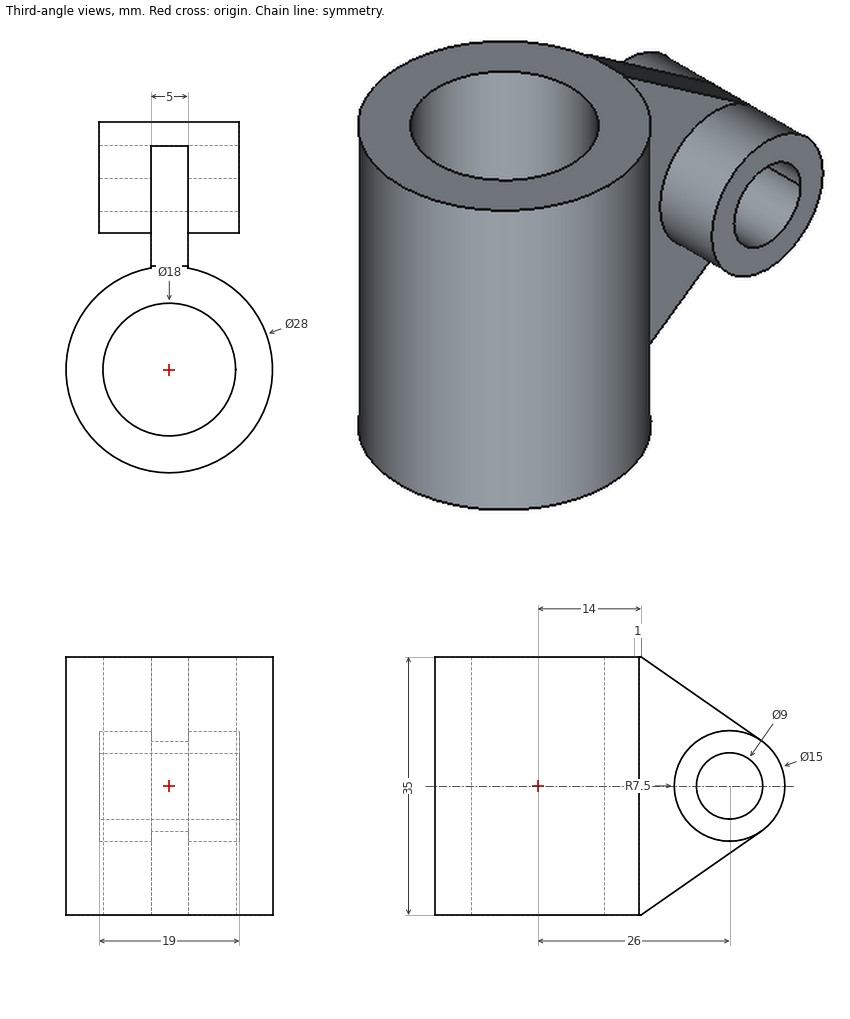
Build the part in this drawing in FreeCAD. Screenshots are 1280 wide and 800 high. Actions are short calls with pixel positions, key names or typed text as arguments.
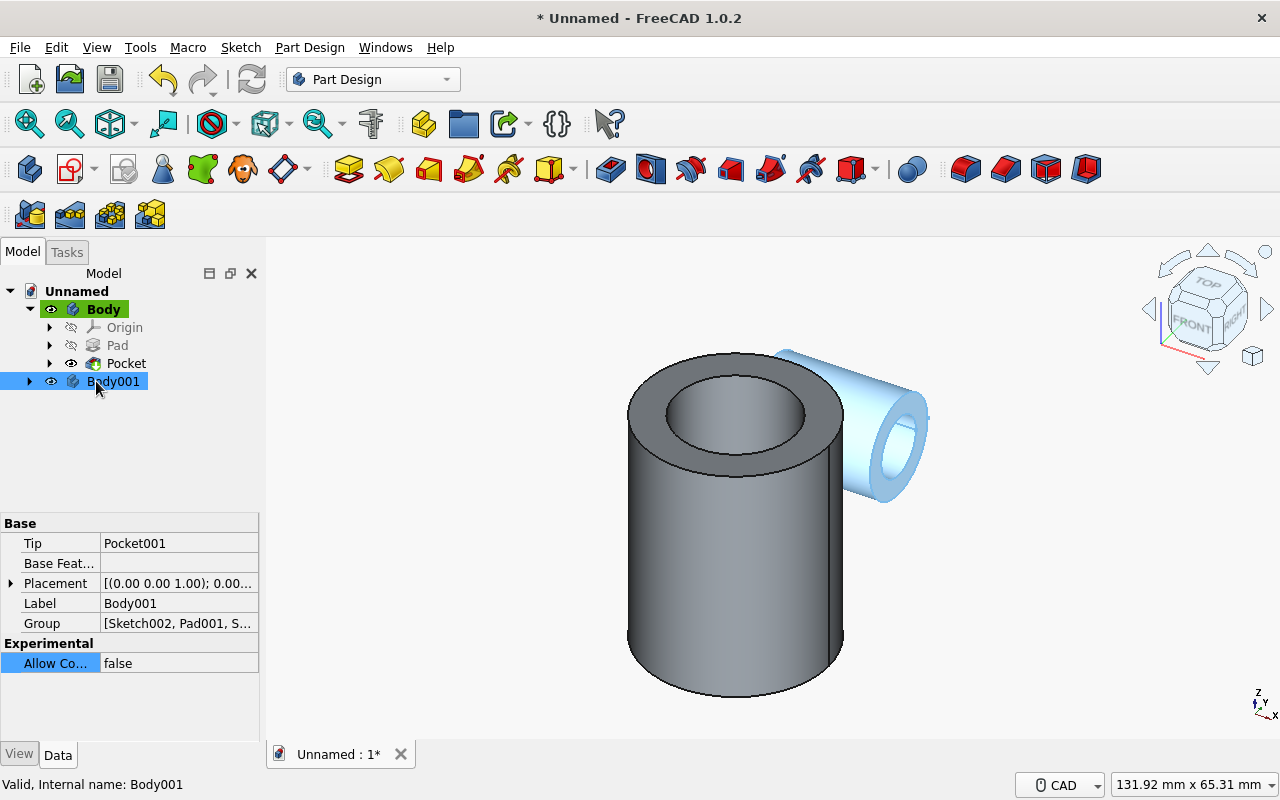
click(914, 170)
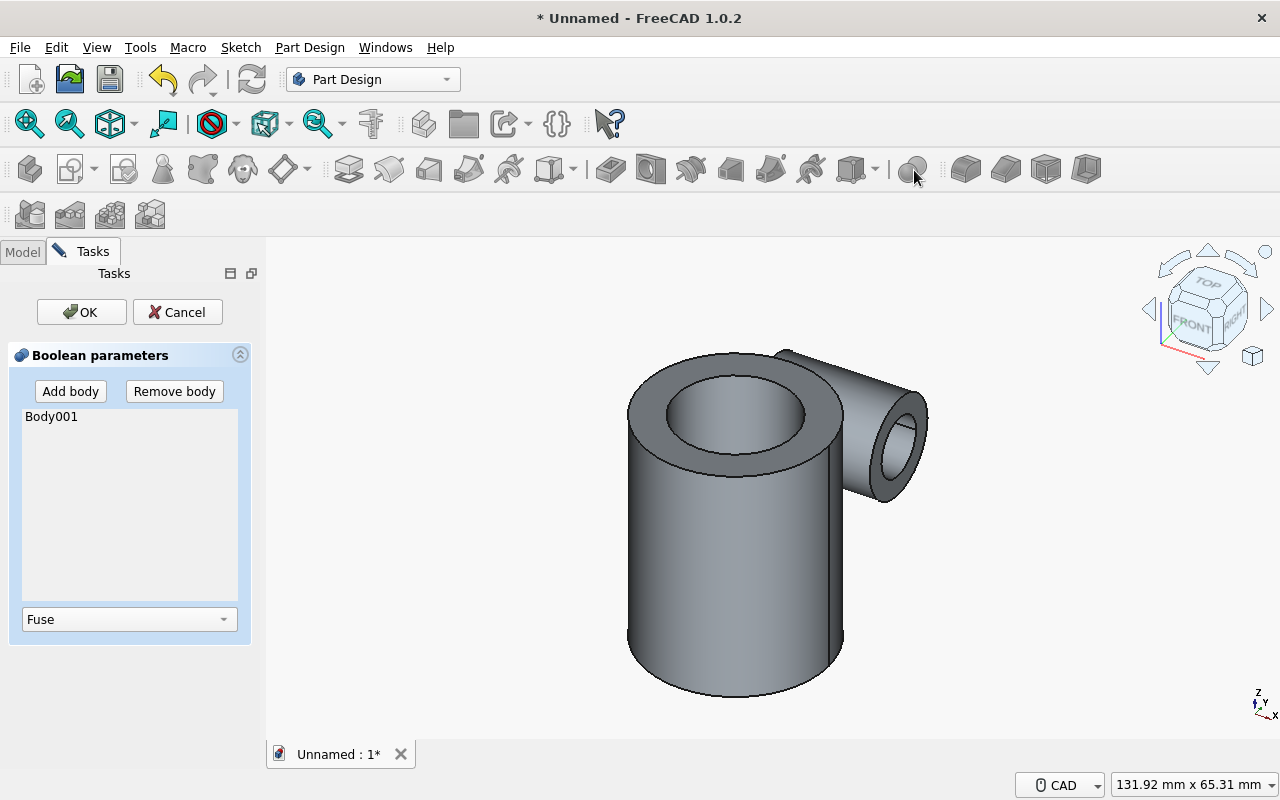
click(82, 312)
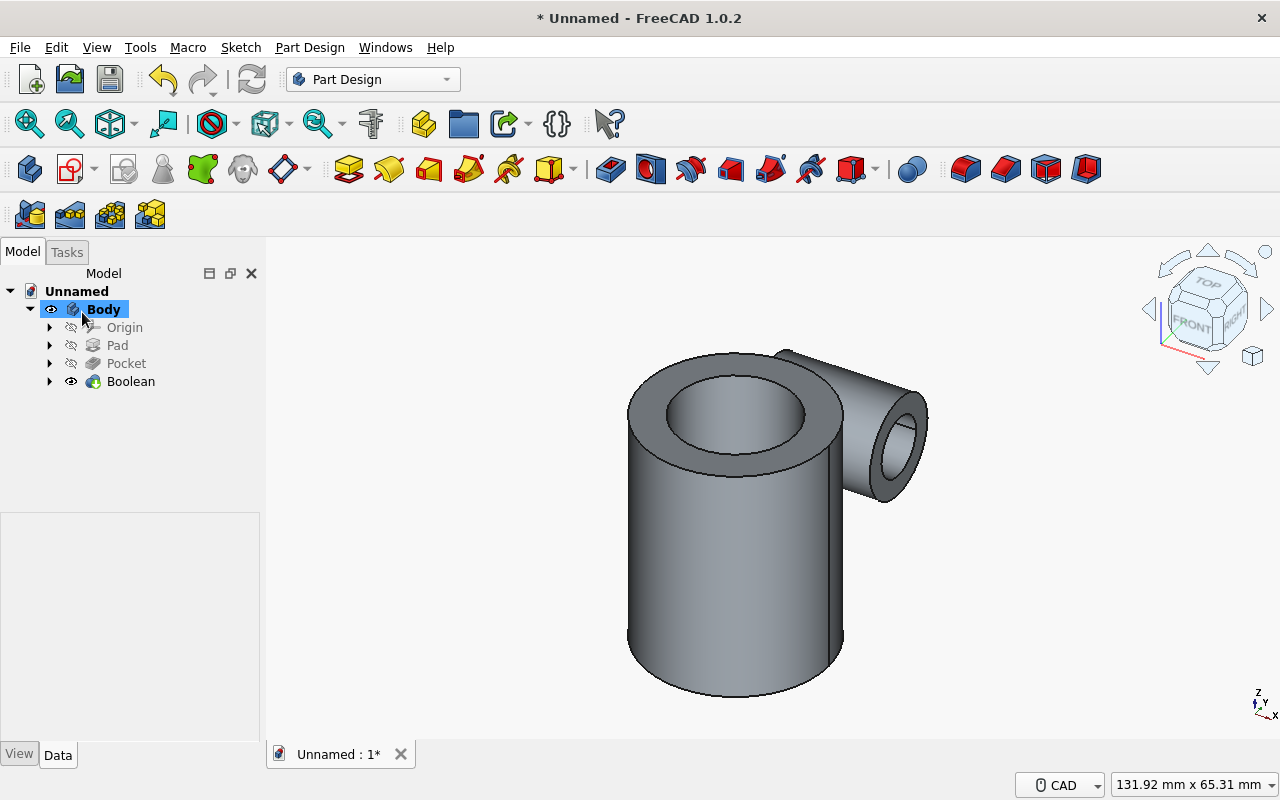
click(70, 170)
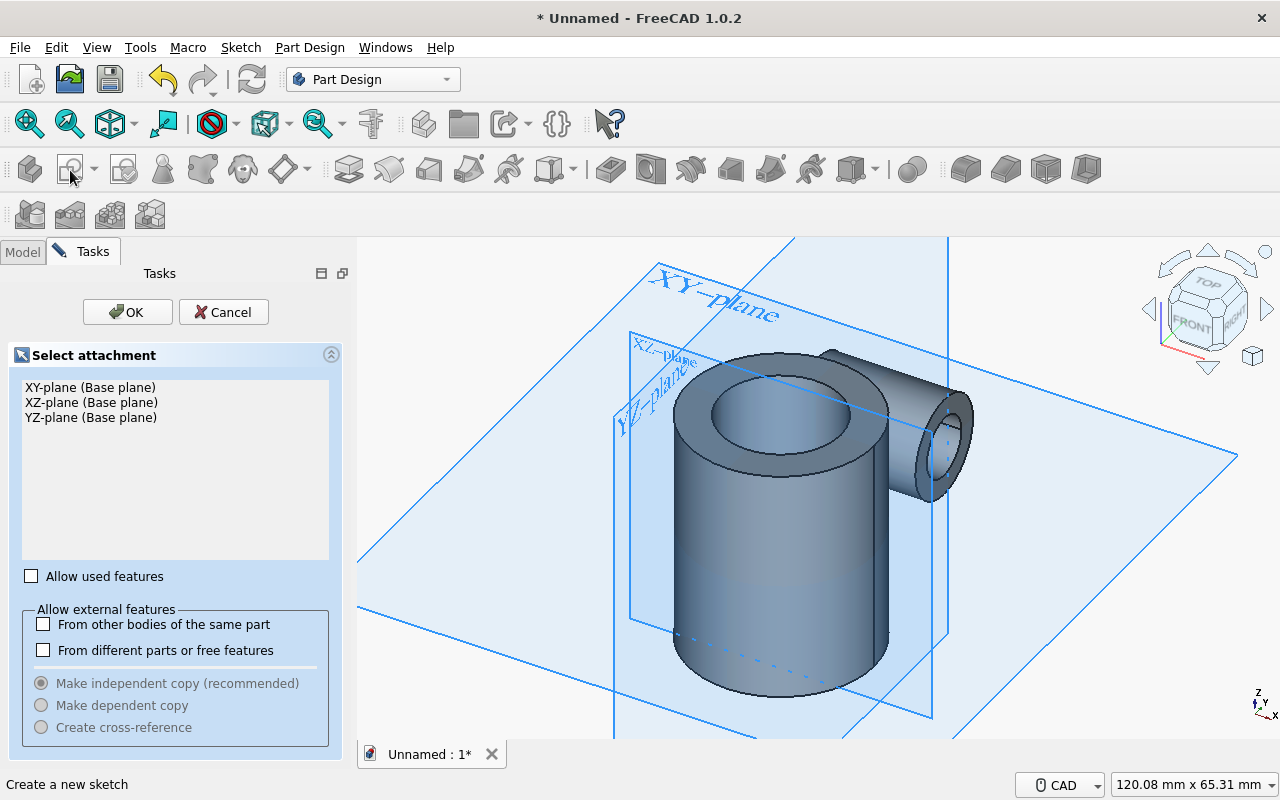
click(82, 418)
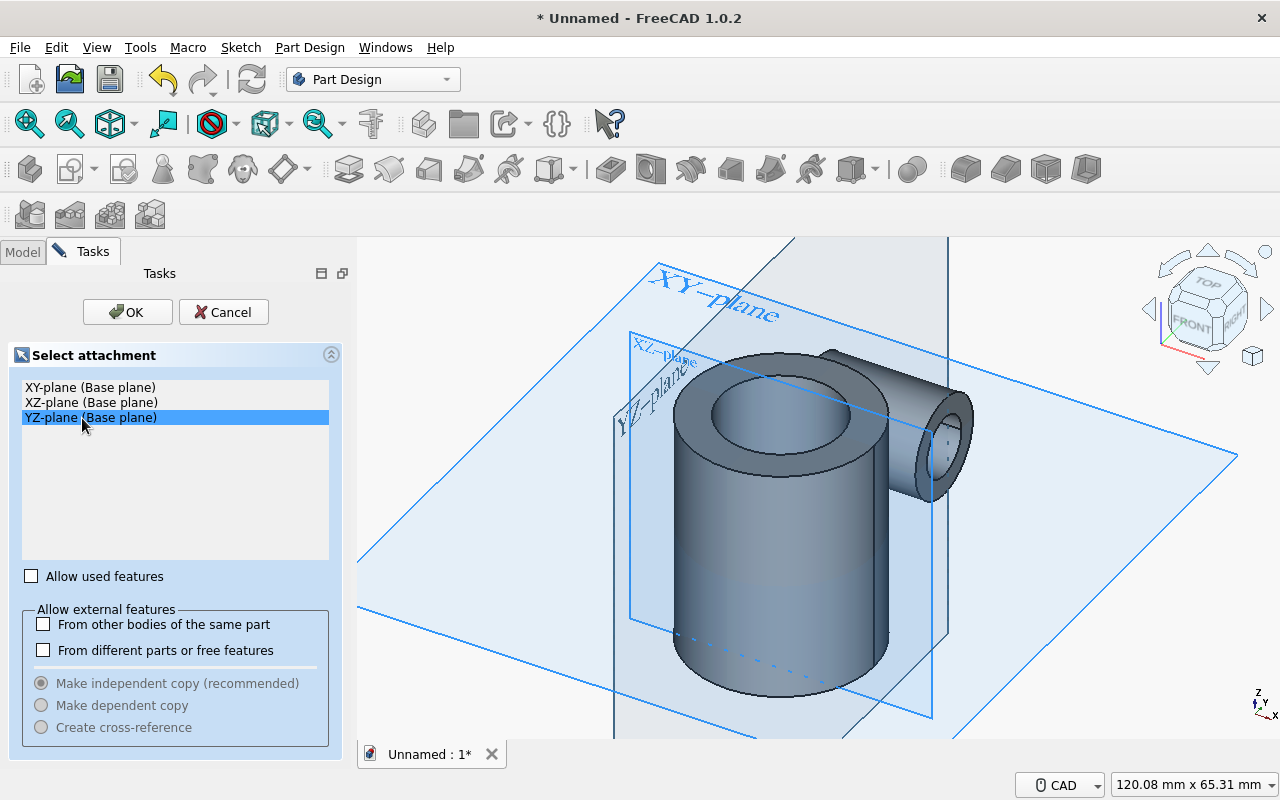
click(128, 312)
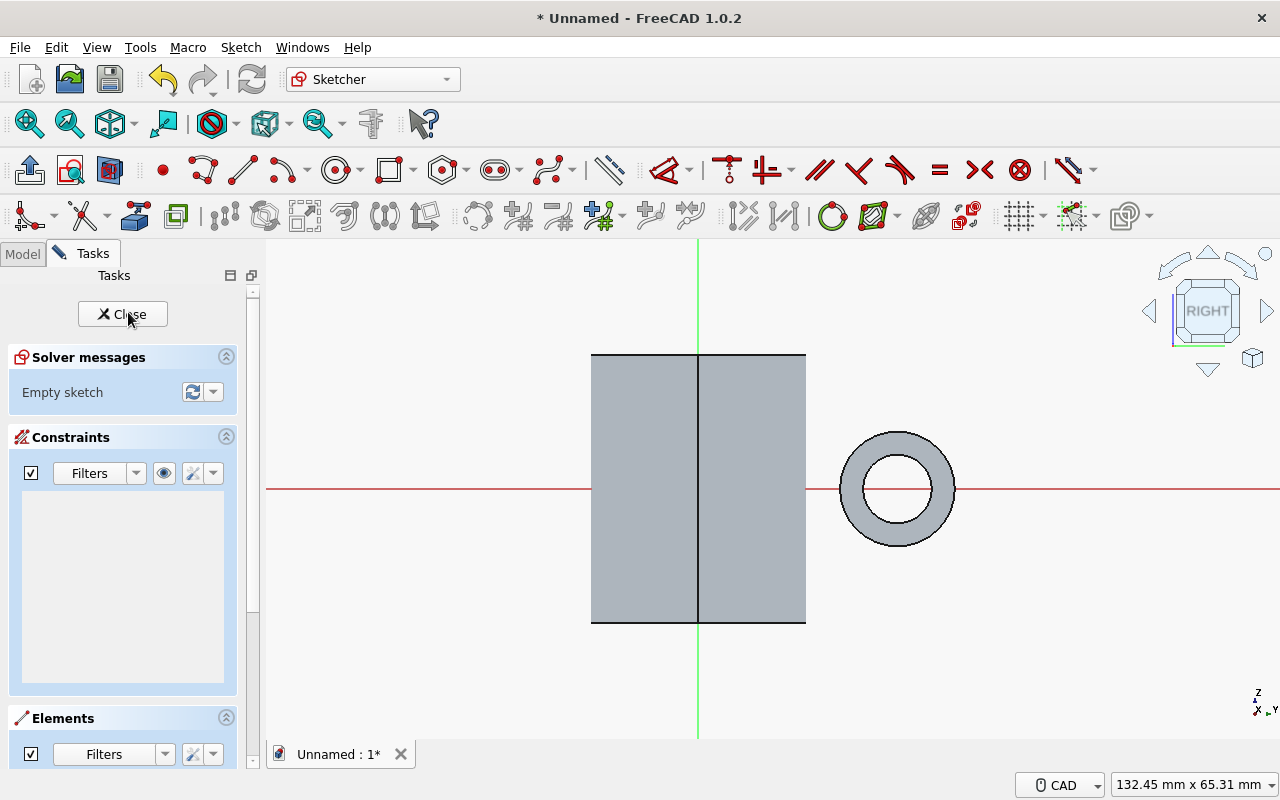
click(110, 170)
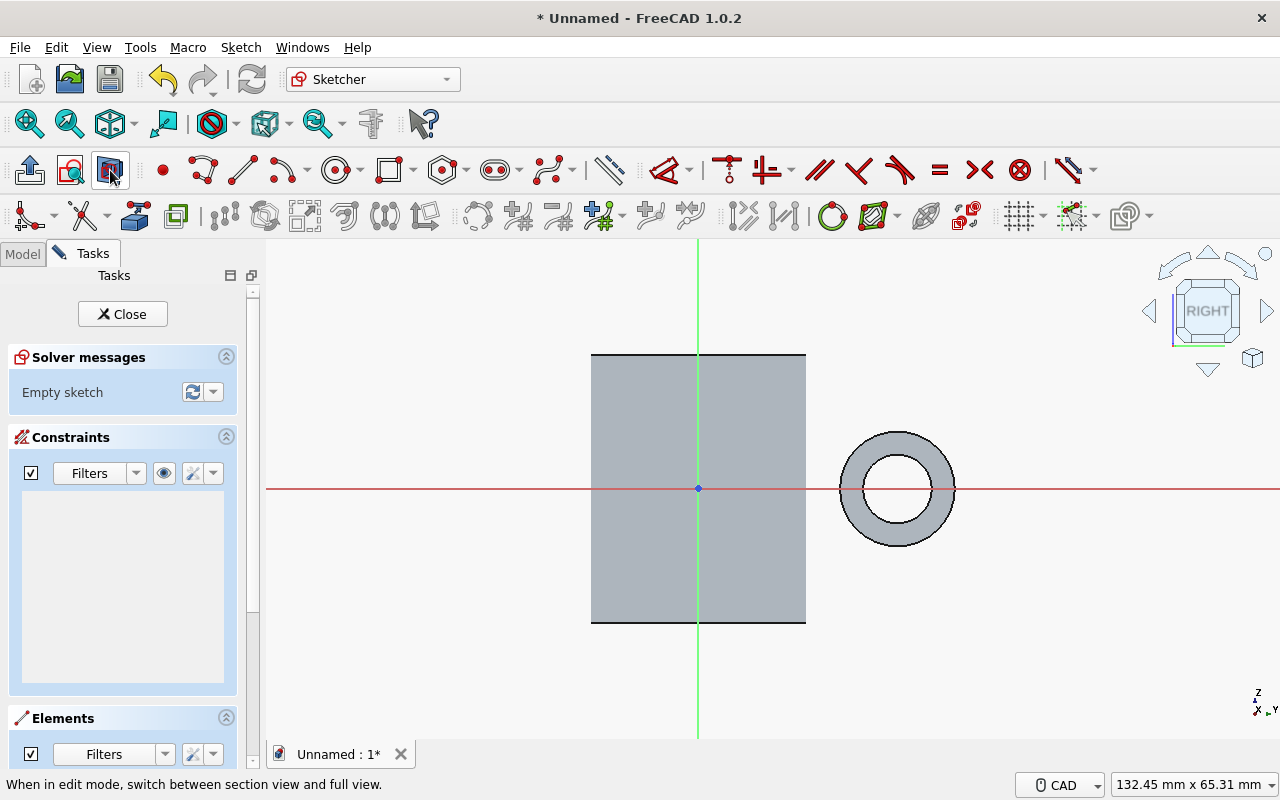
key(g)
key(m)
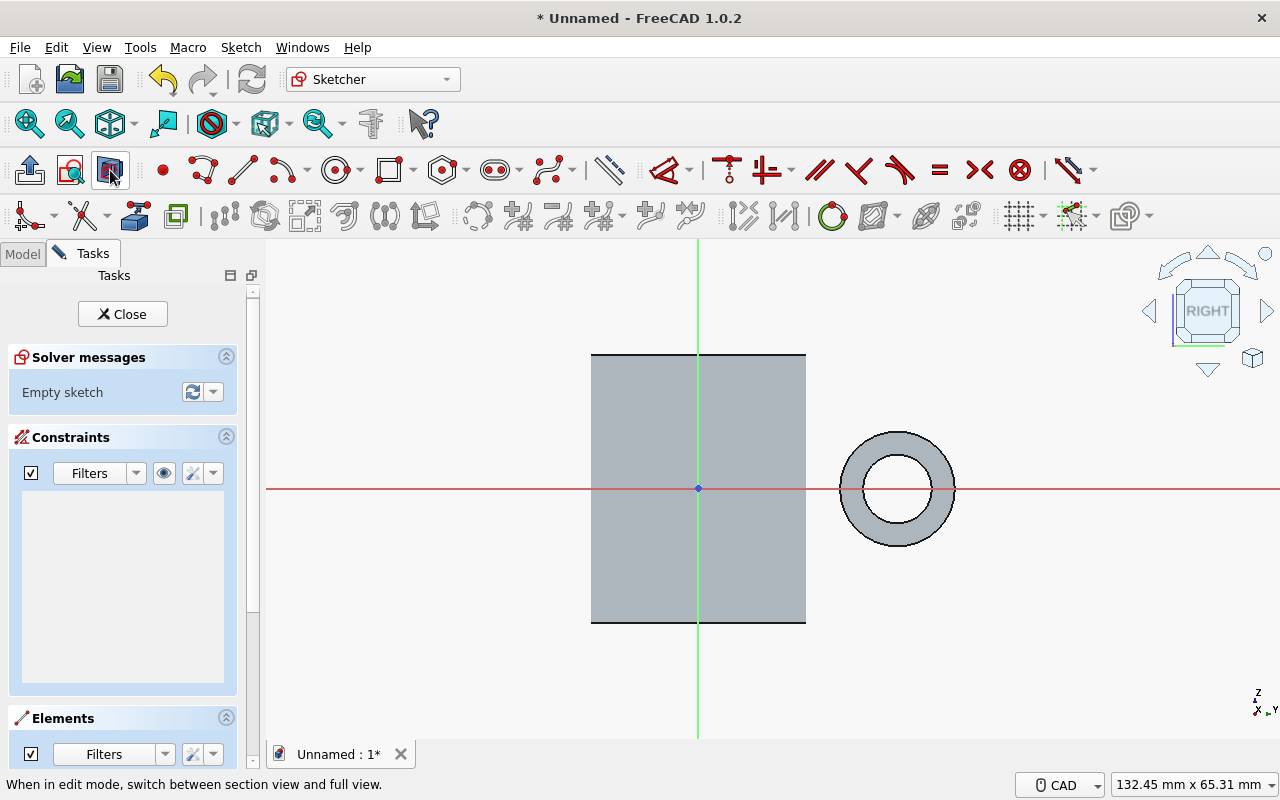
click(930, 442)
click(806, 355)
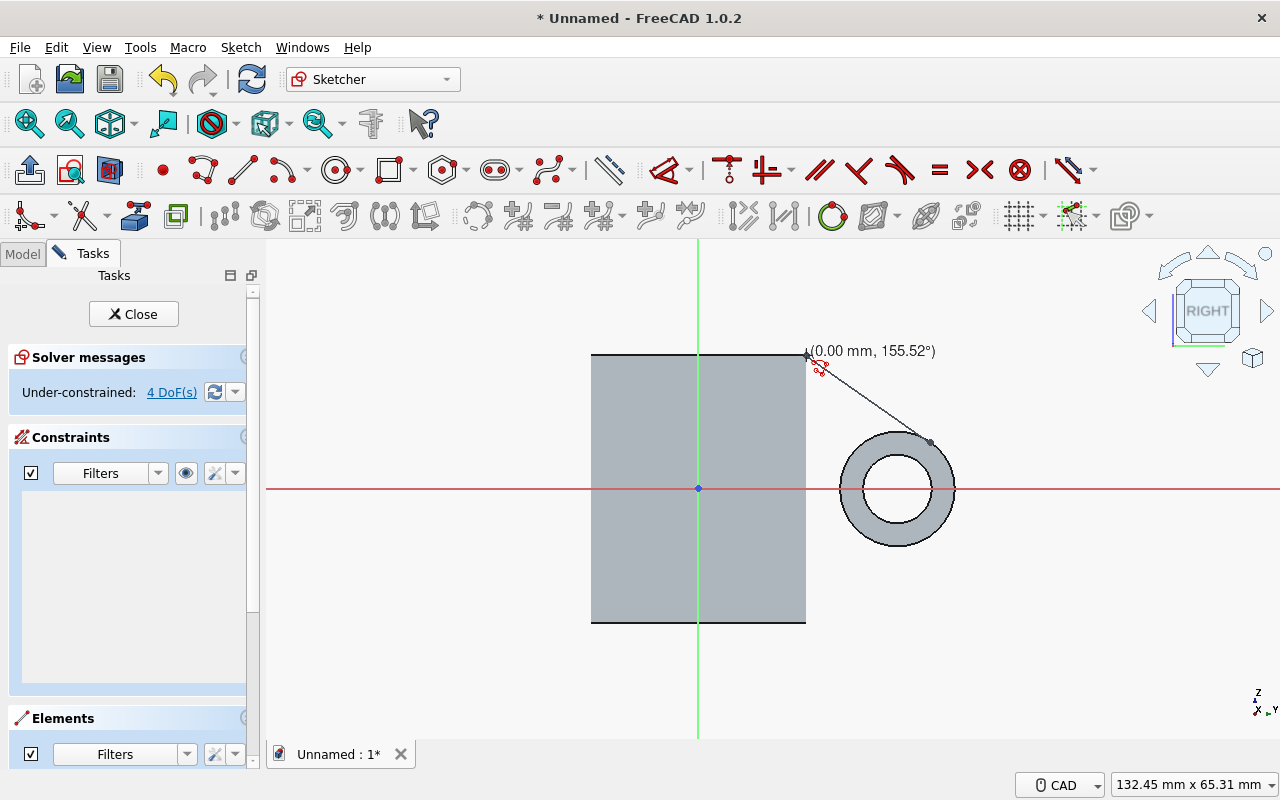
scroll(798, 355, up, 4)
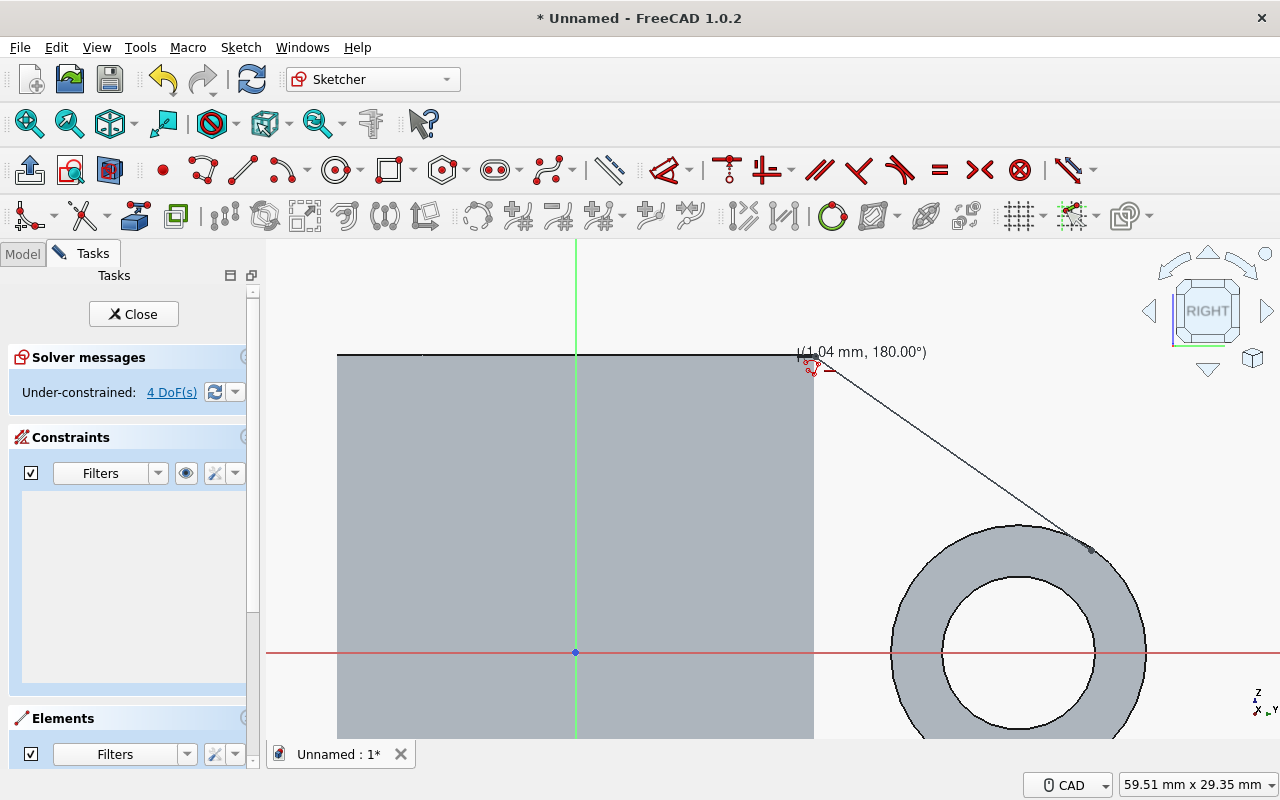
click(797, 355)